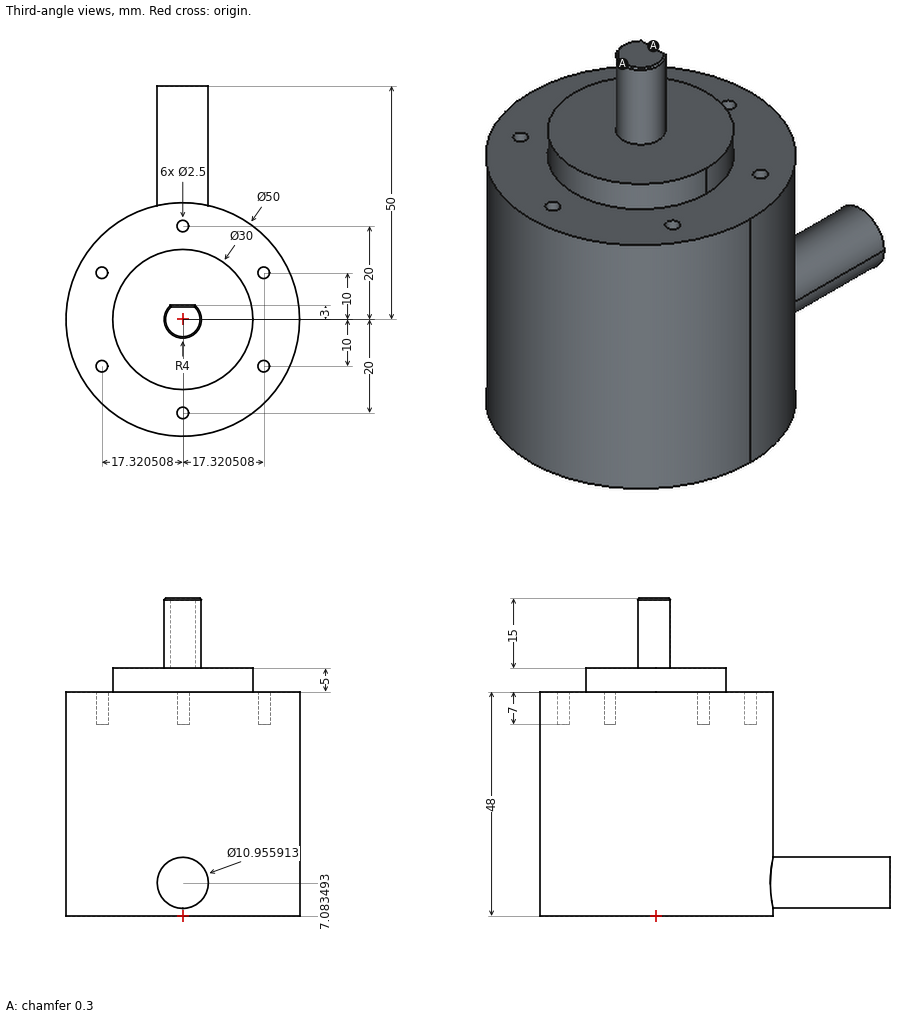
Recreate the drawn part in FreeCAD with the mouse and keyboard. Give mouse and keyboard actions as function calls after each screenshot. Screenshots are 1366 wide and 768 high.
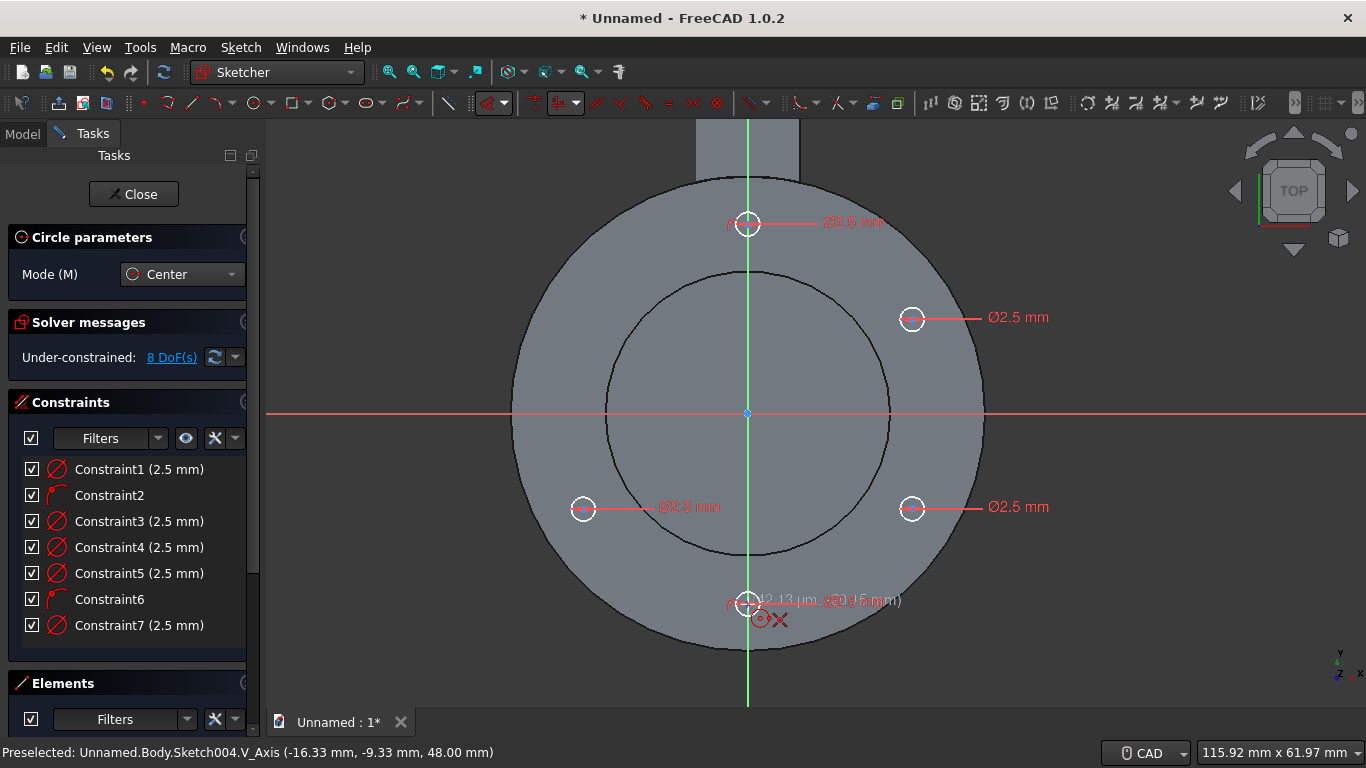
scroll(583, 319, up, 4)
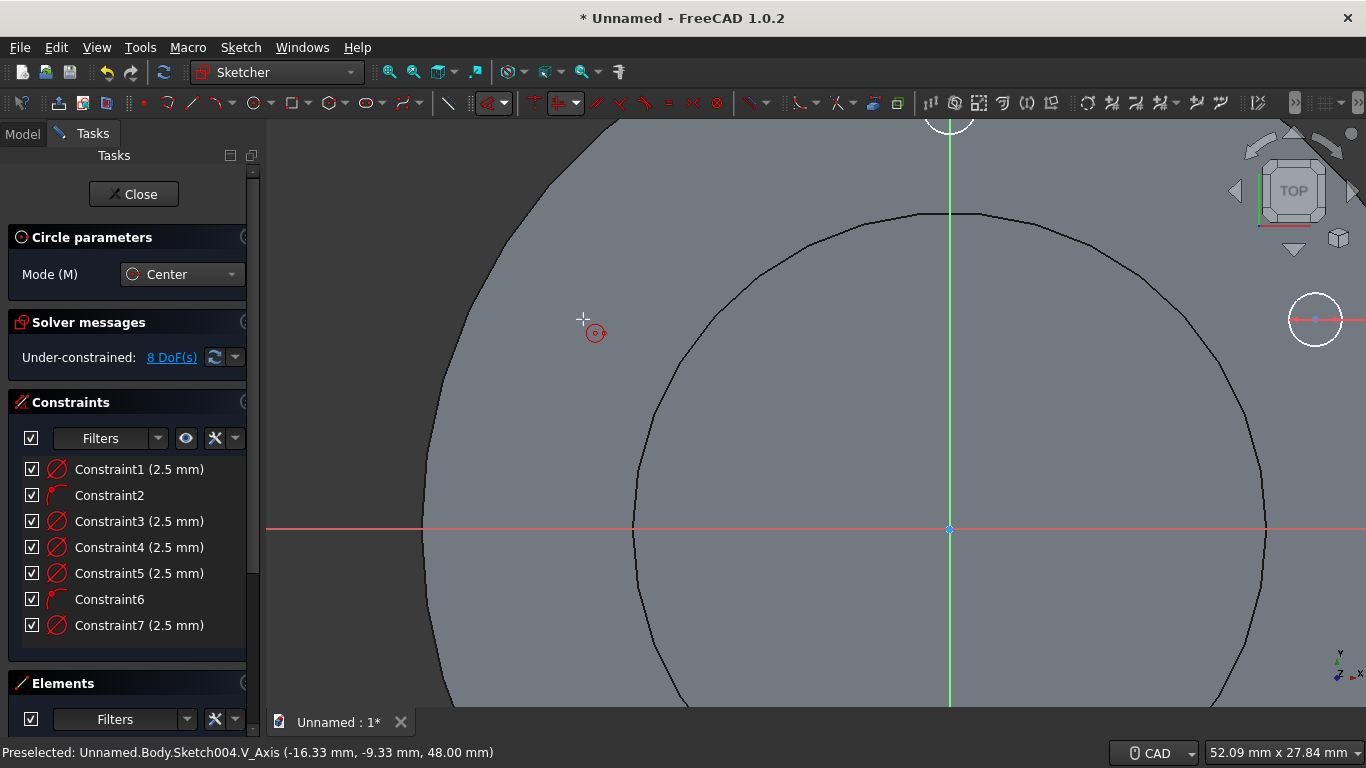
click(584, 318)
move(602, 300)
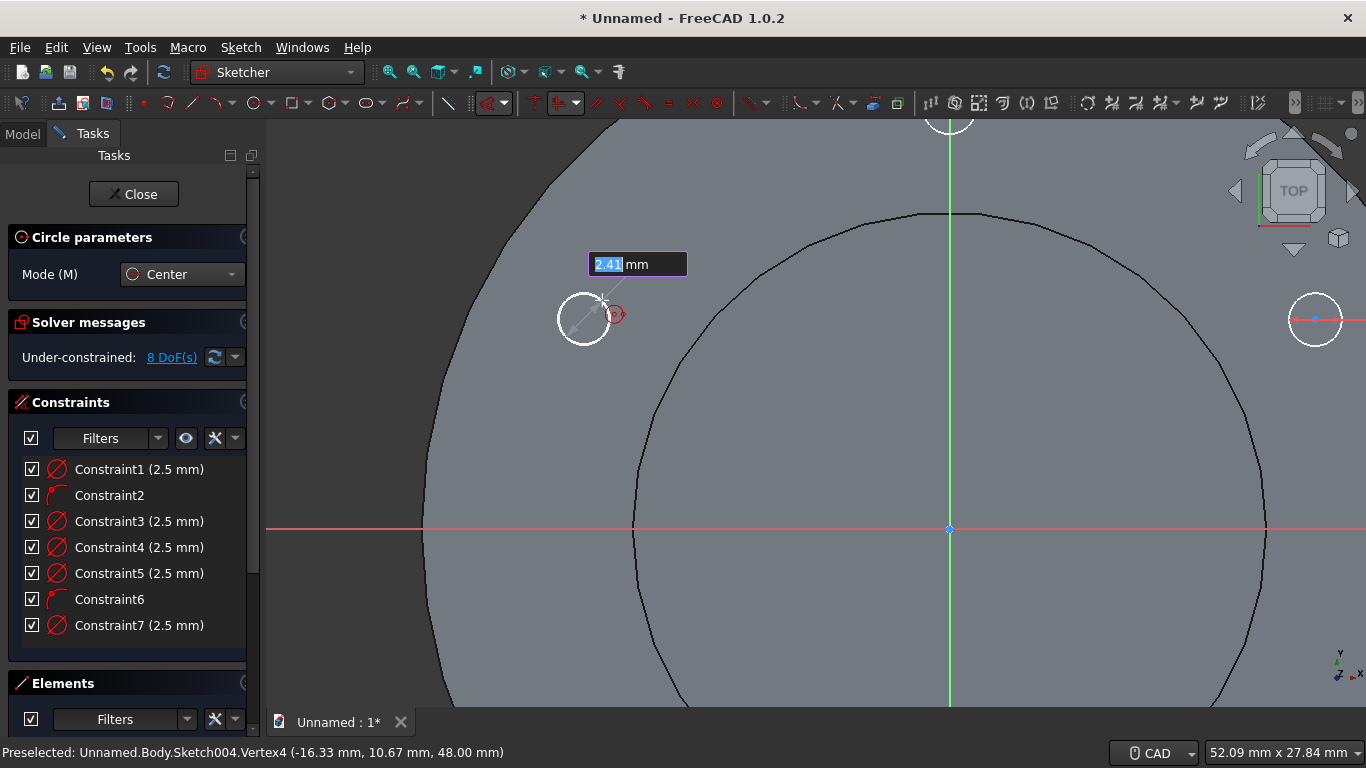
text(2.5)
key(Return)
key(Escape)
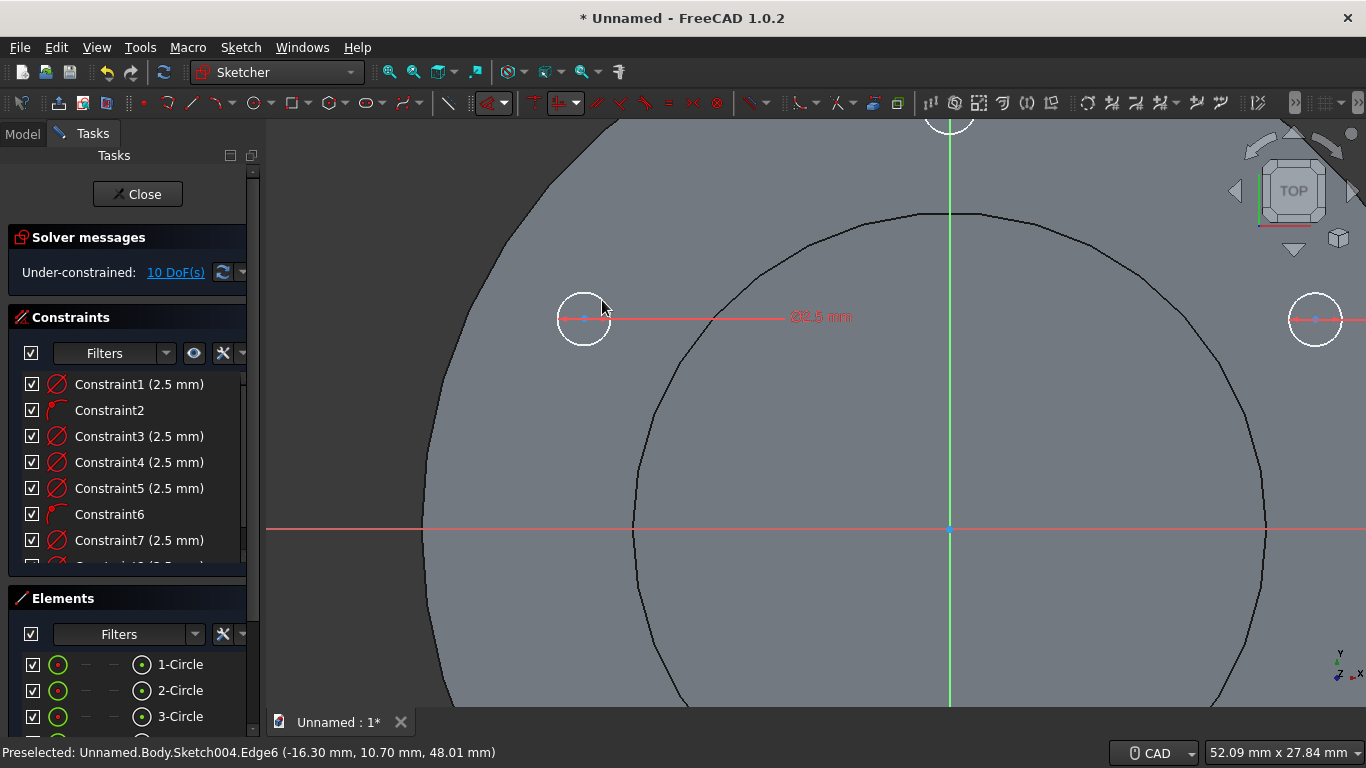
scroll(583, 318, down, 4)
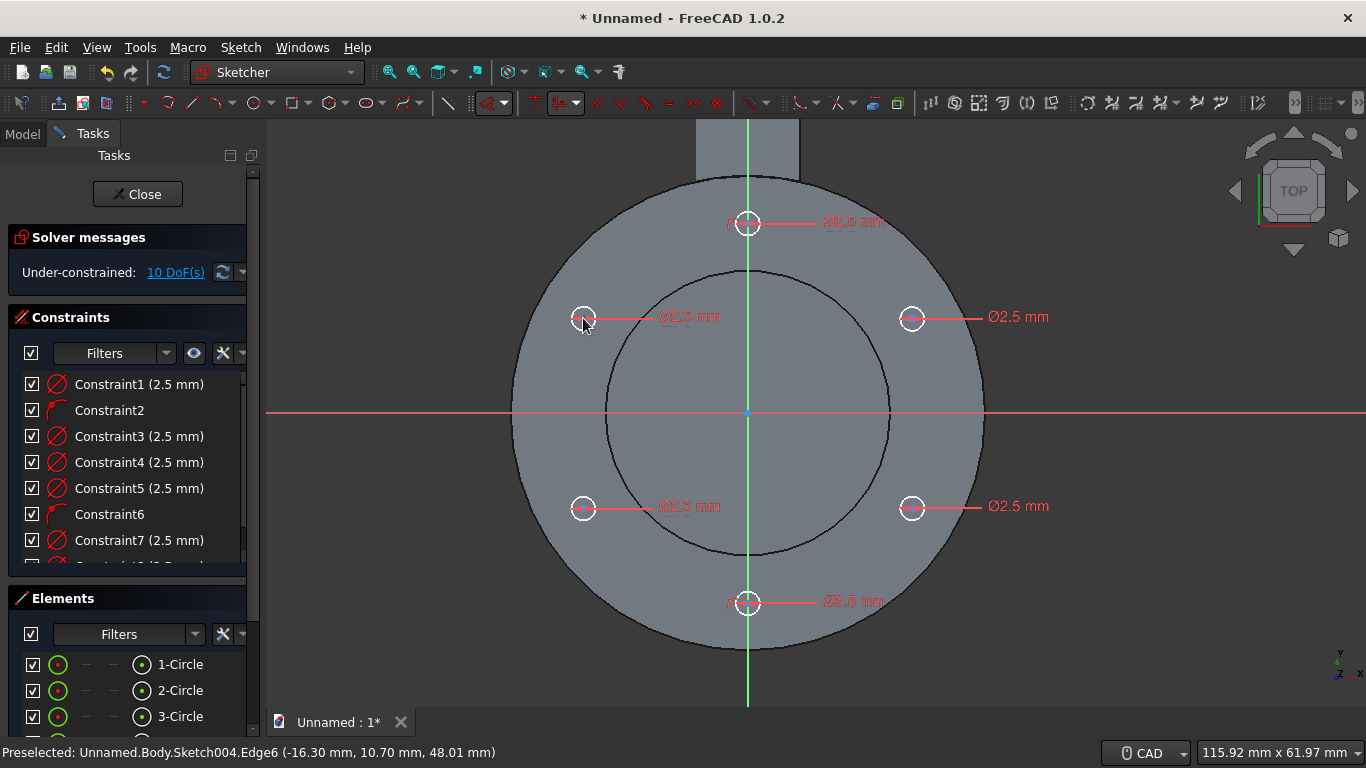
click(912, 319)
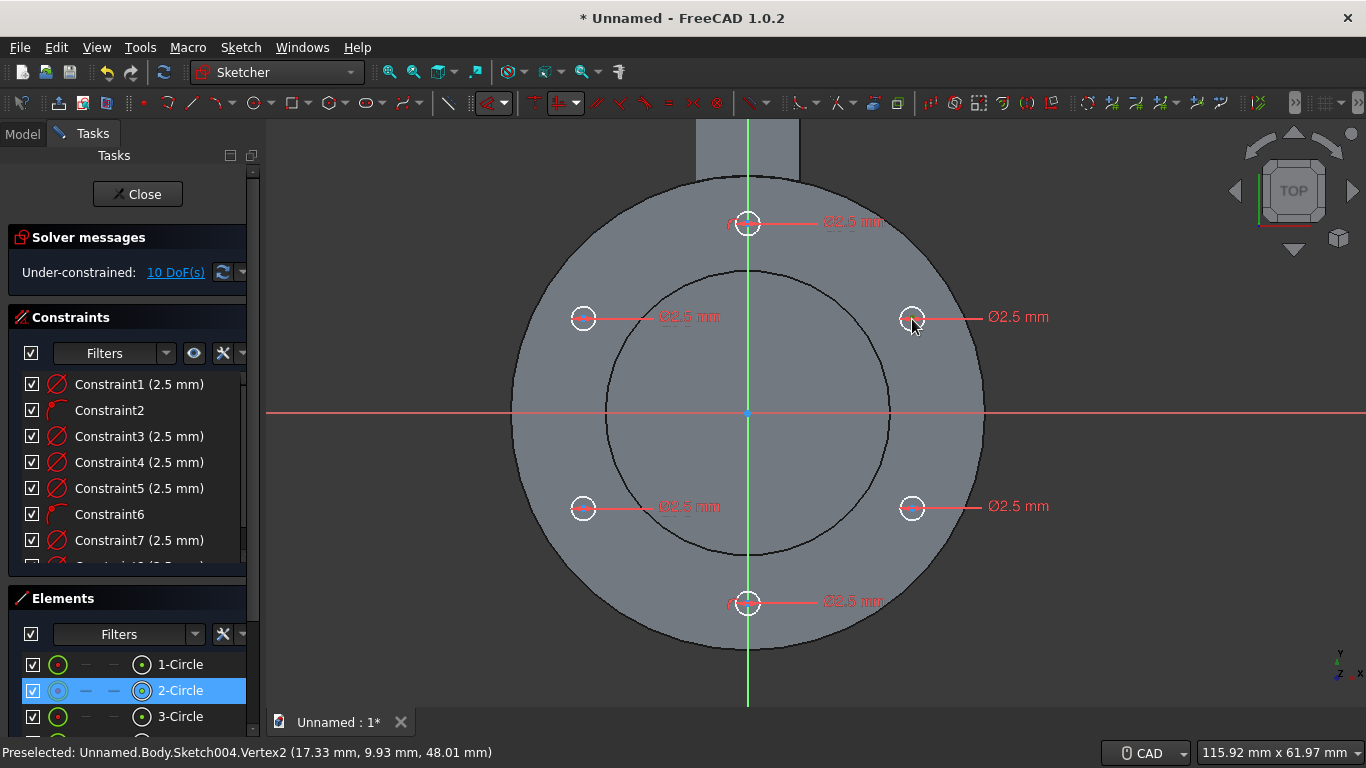
click(912, 508)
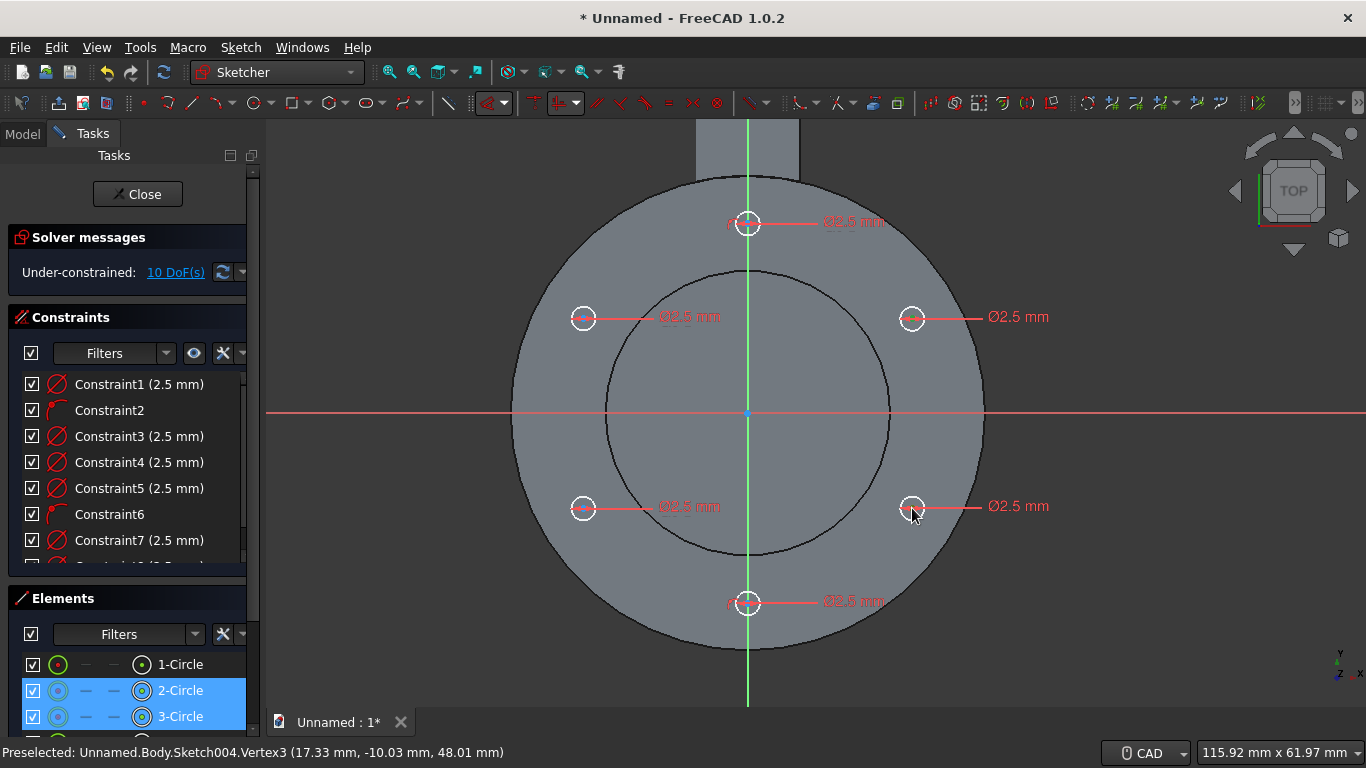
key(v)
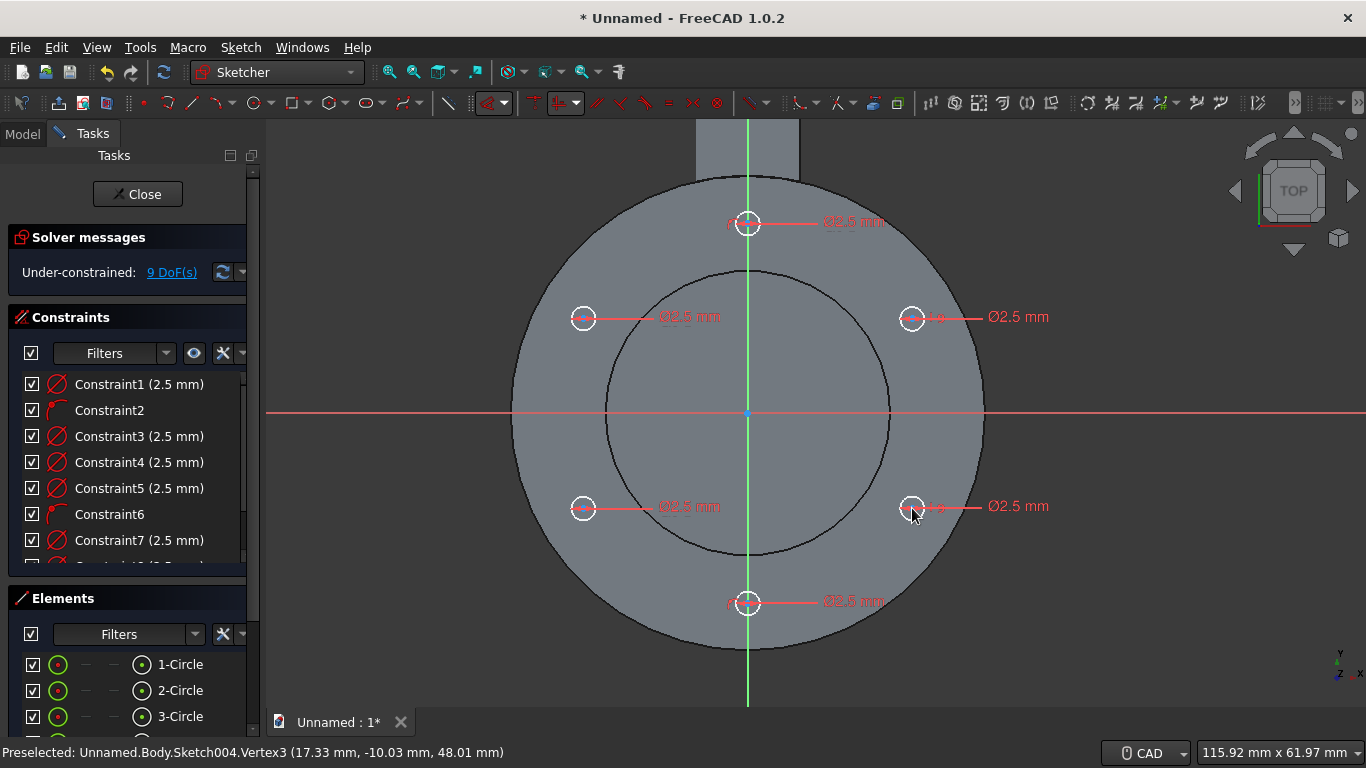
click(912, 508)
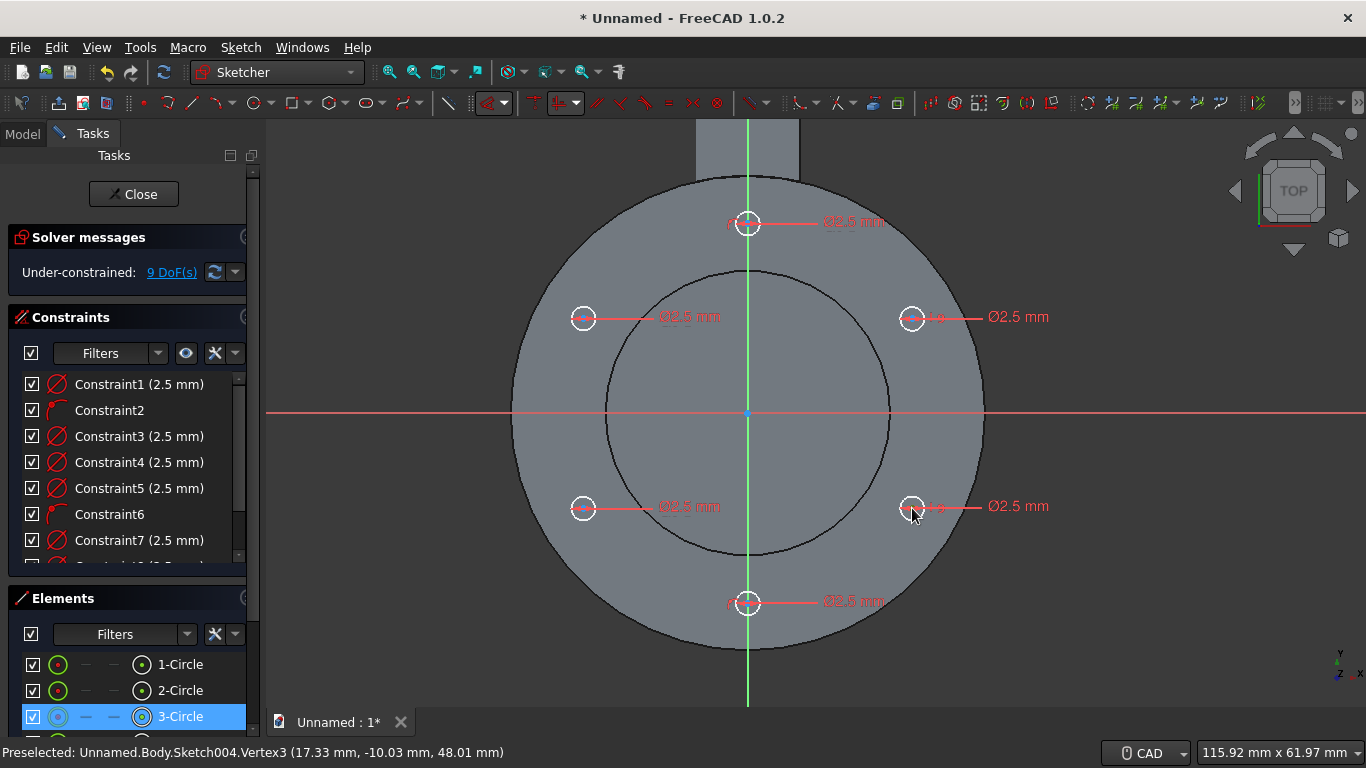
click(583, 509)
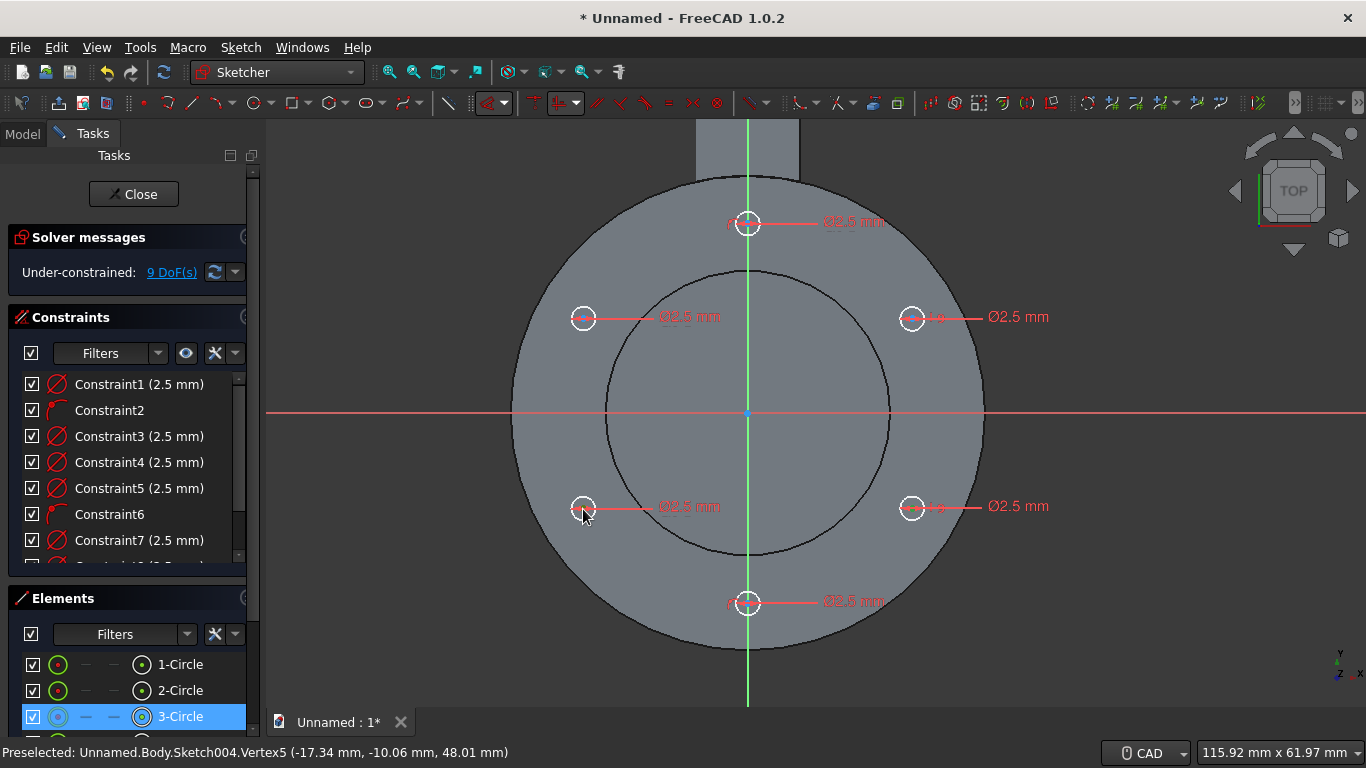
key(h)